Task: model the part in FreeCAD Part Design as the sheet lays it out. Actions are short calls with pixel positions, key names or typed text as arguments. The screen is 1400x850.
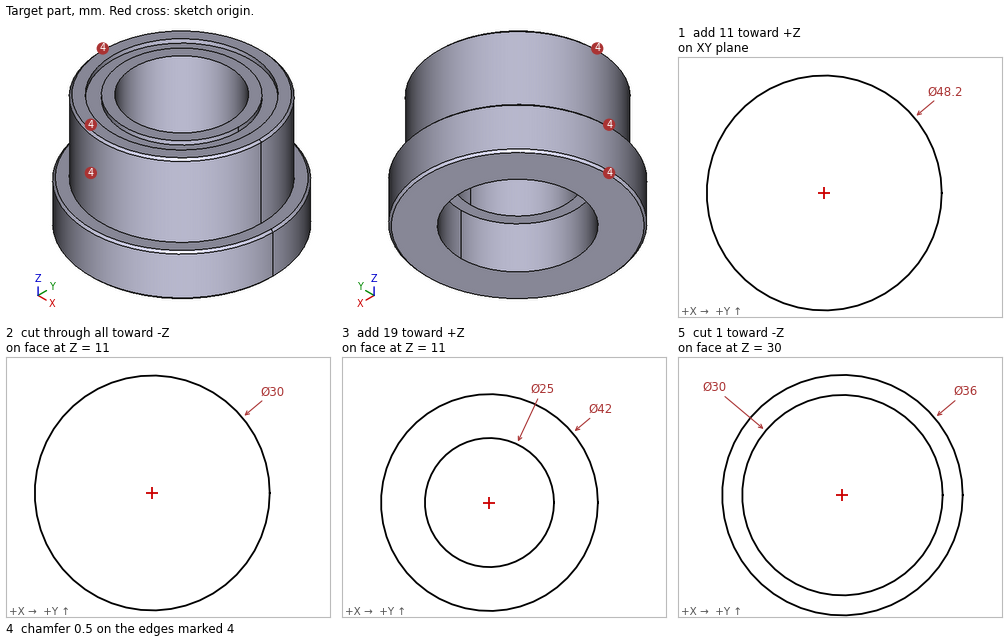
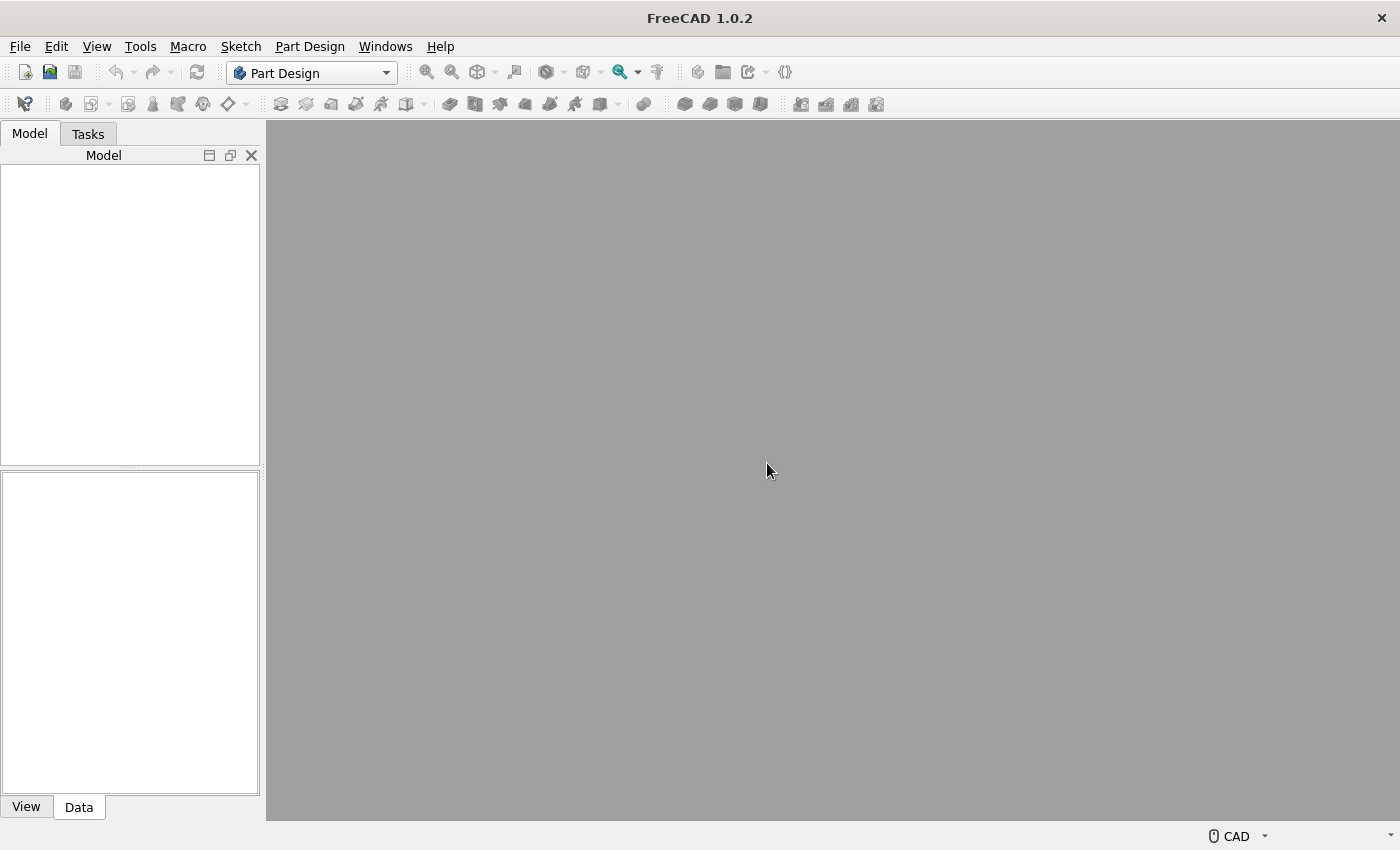
key(ctrl+n)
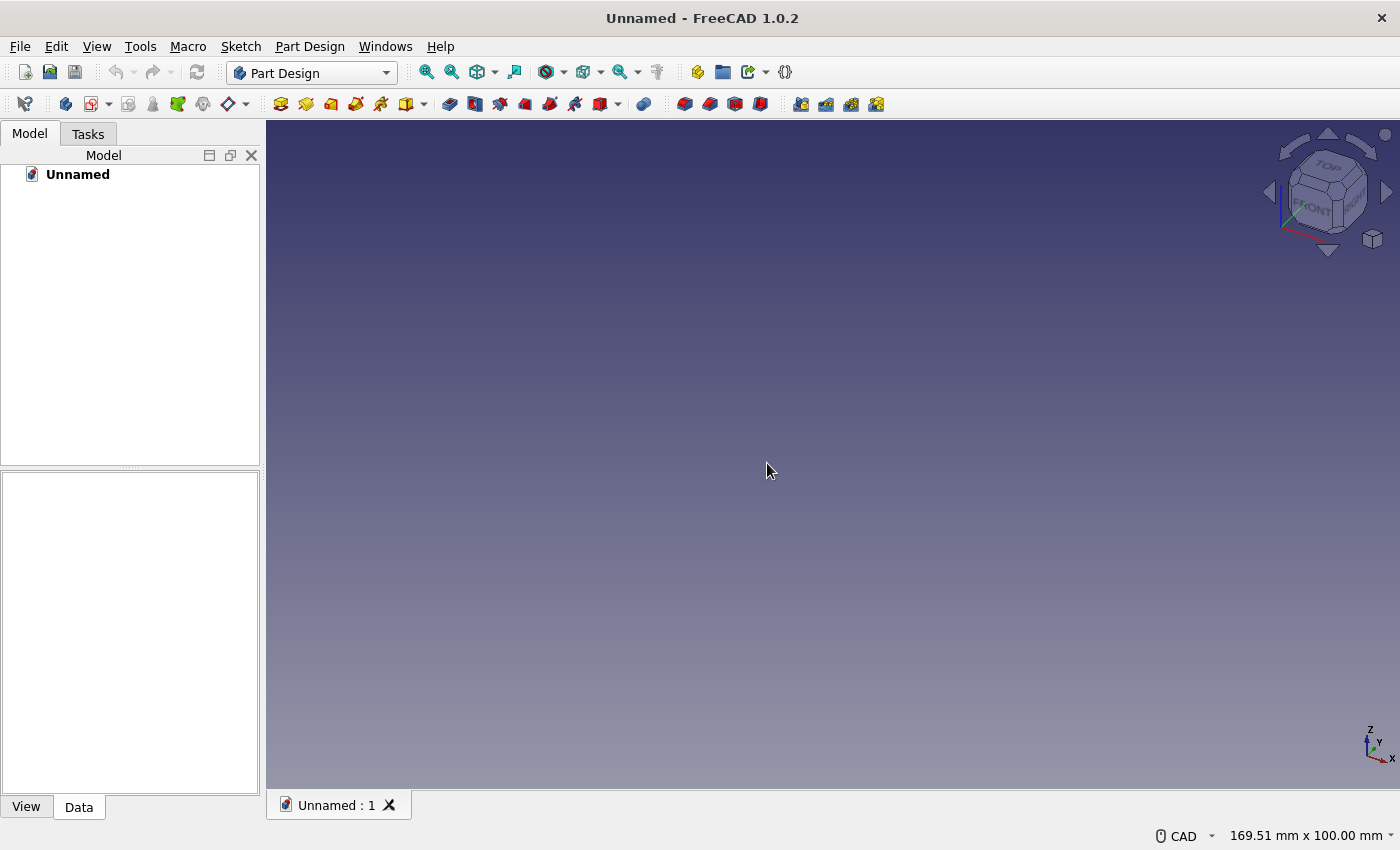
click(90, 104)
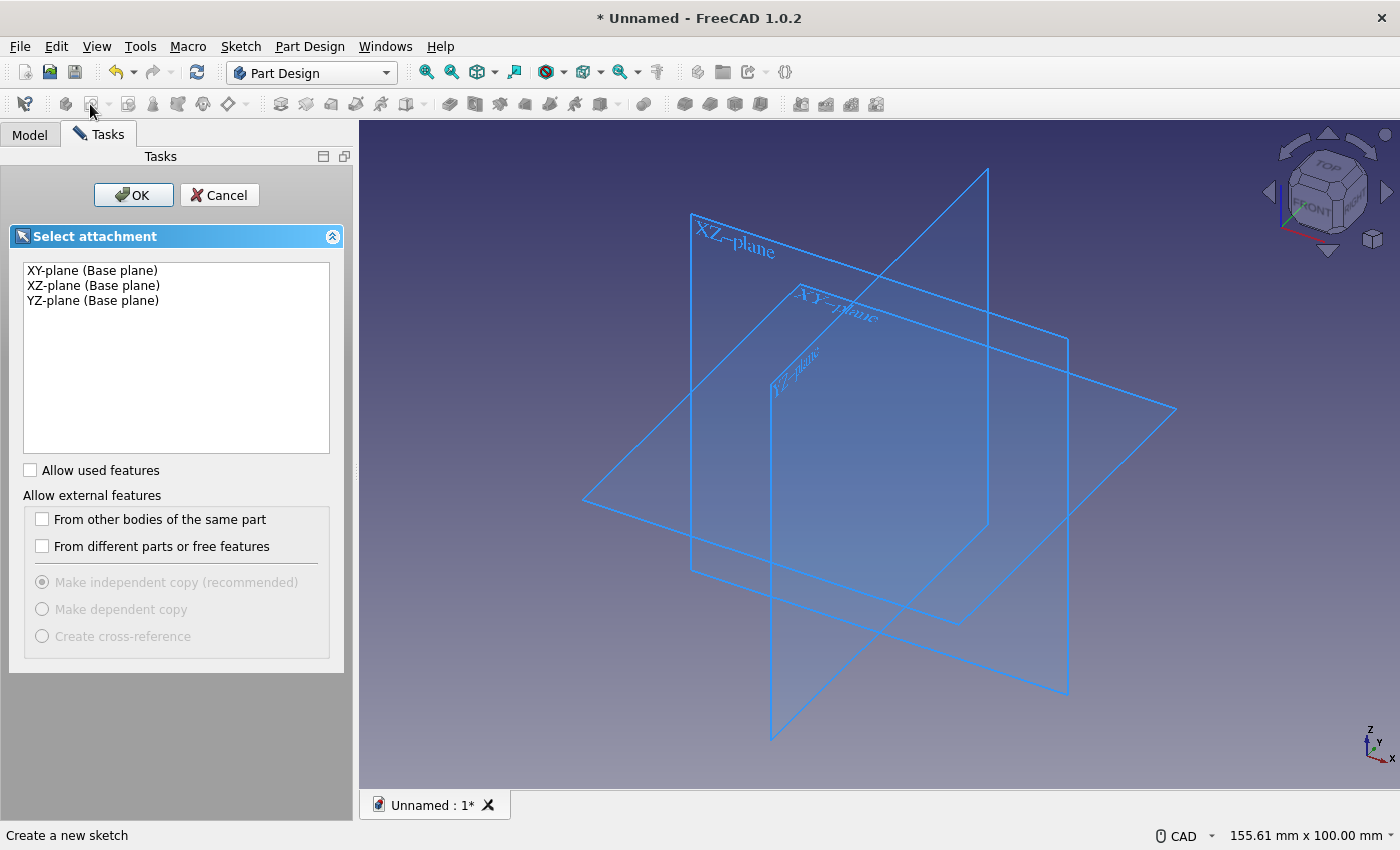
click(84, 270)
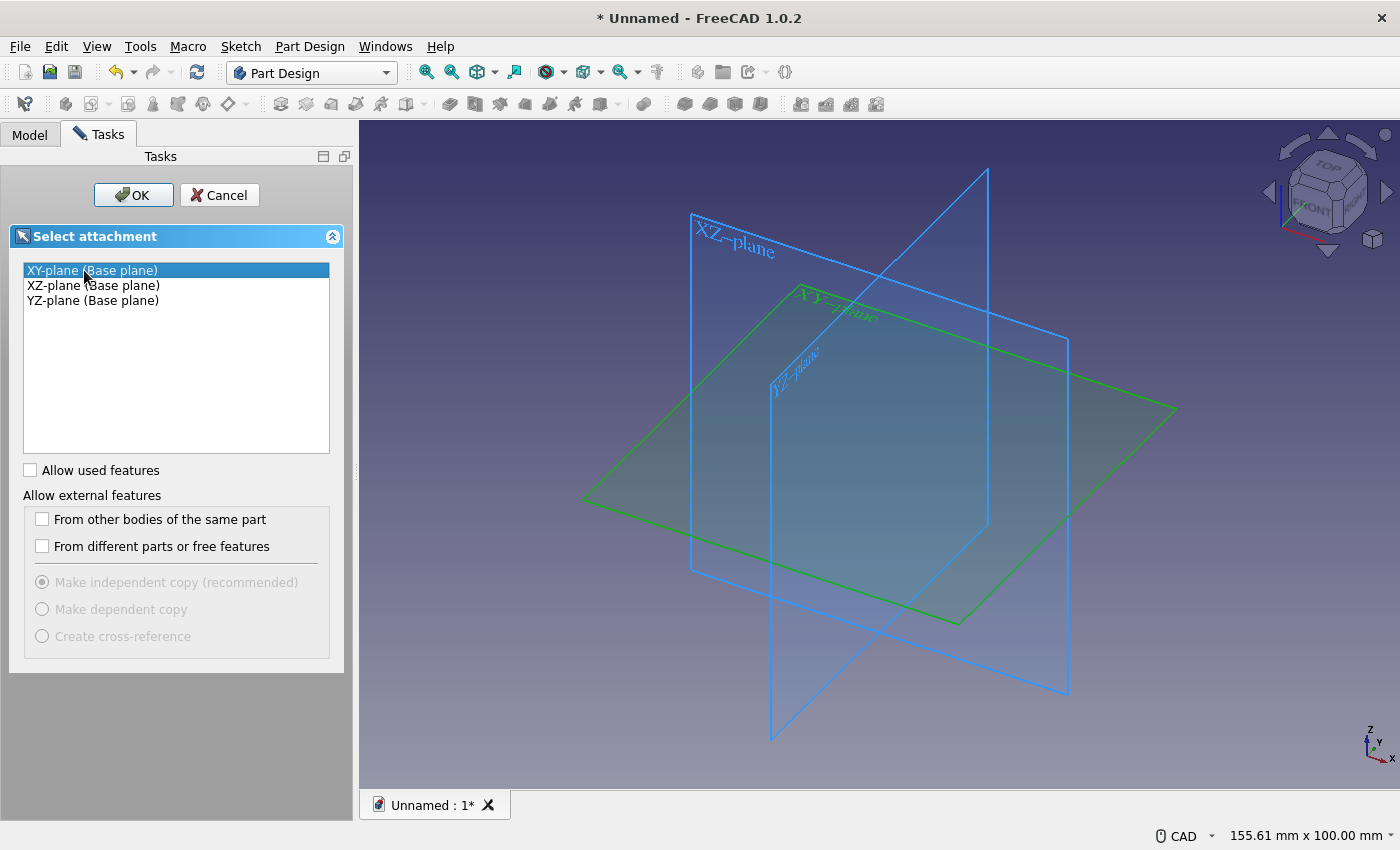
click(134, 195)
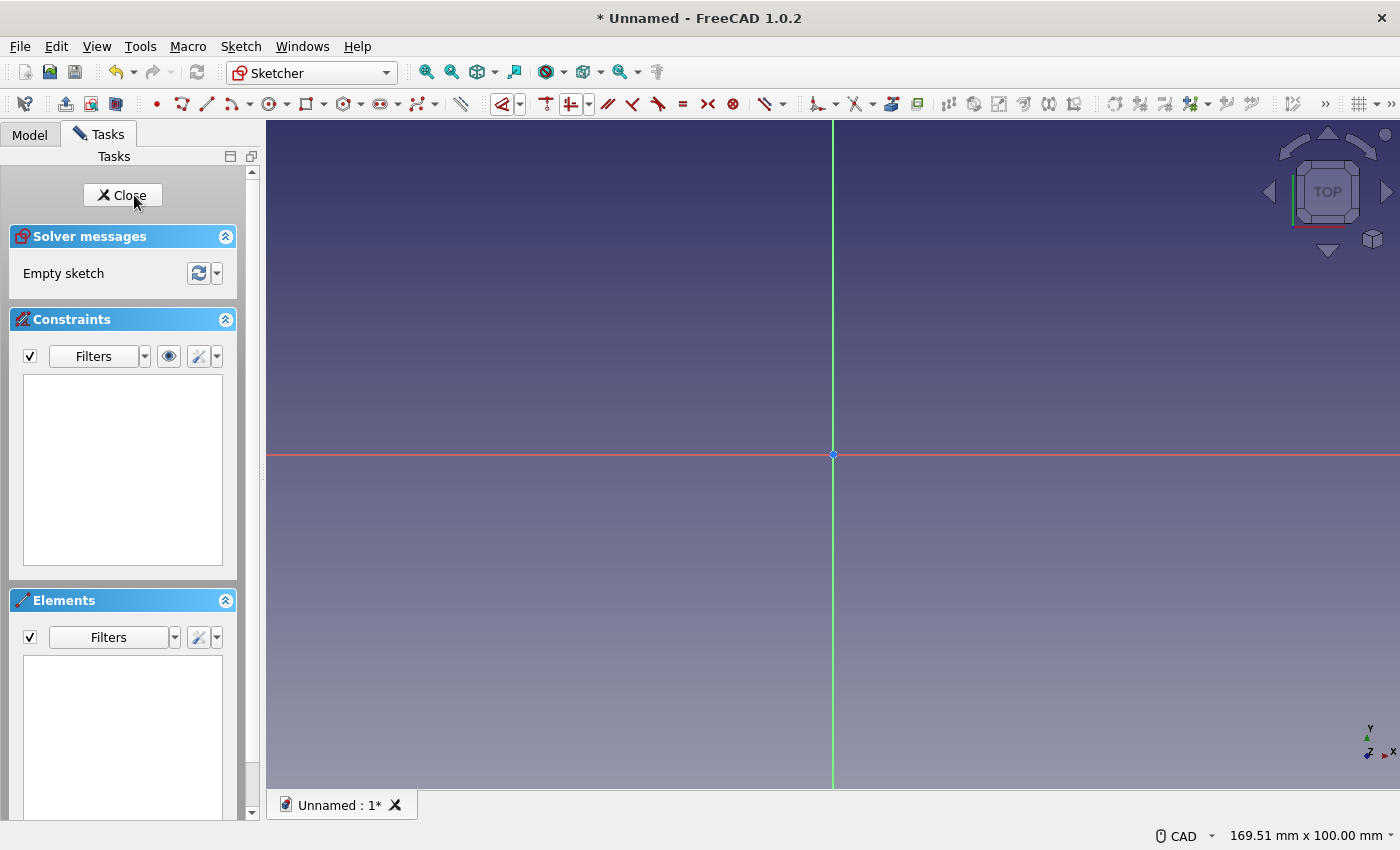
click(268, 104)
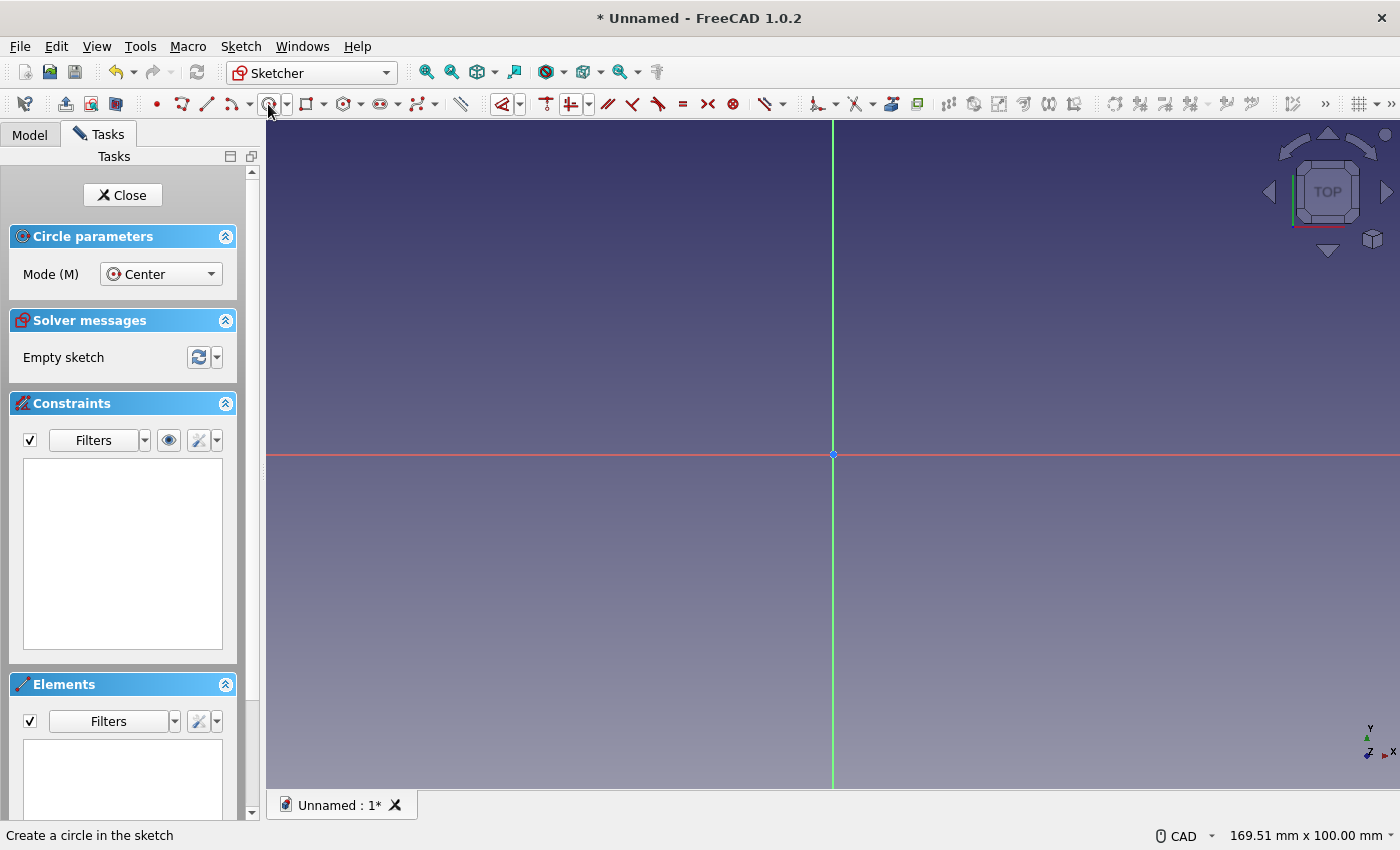
click(833, 454)
click(947, 340)
key(Escape)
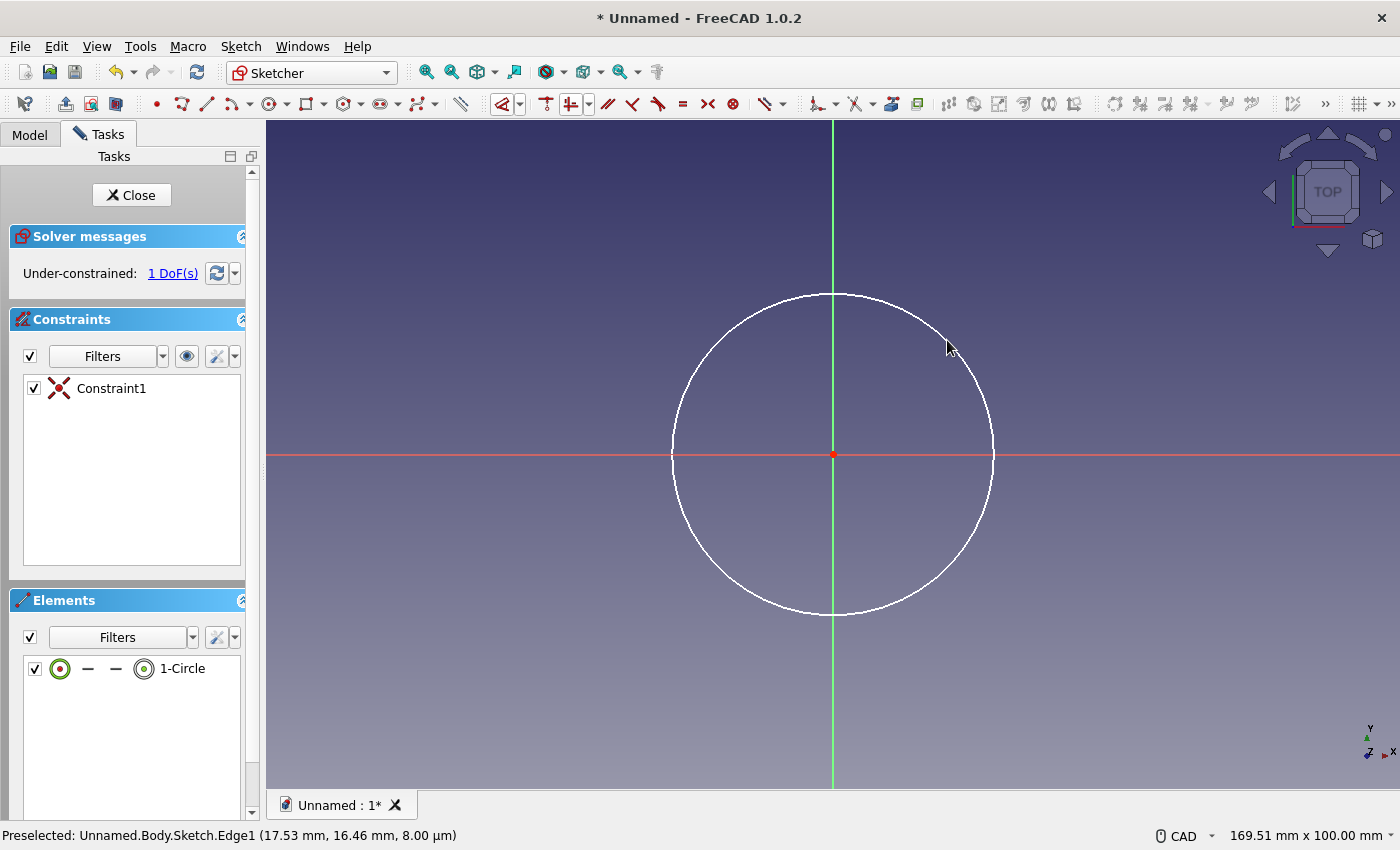
key(d)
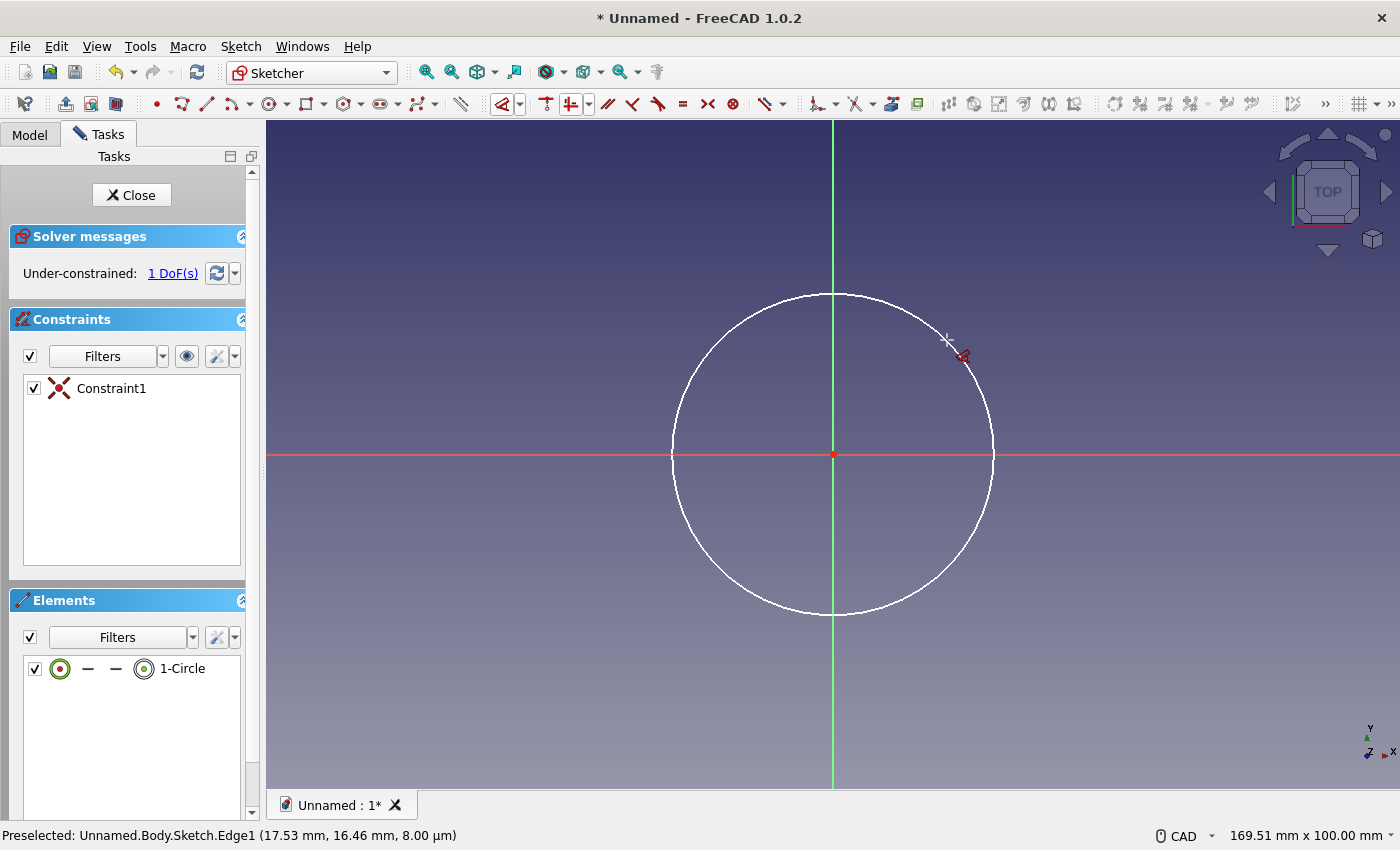
click(946, 340)
click(968, 317)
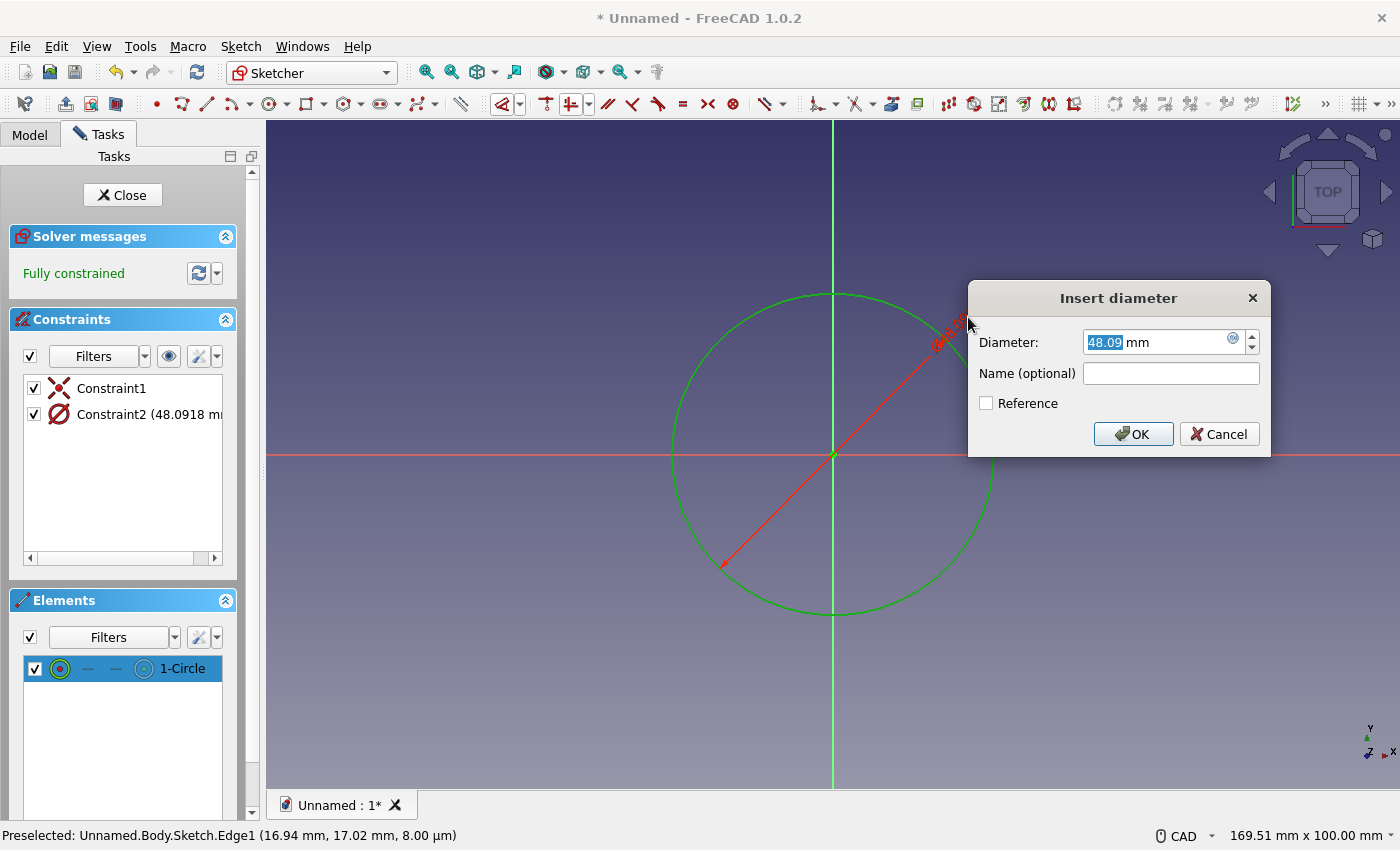
text(48.2)
key(Return)
key(Escape)